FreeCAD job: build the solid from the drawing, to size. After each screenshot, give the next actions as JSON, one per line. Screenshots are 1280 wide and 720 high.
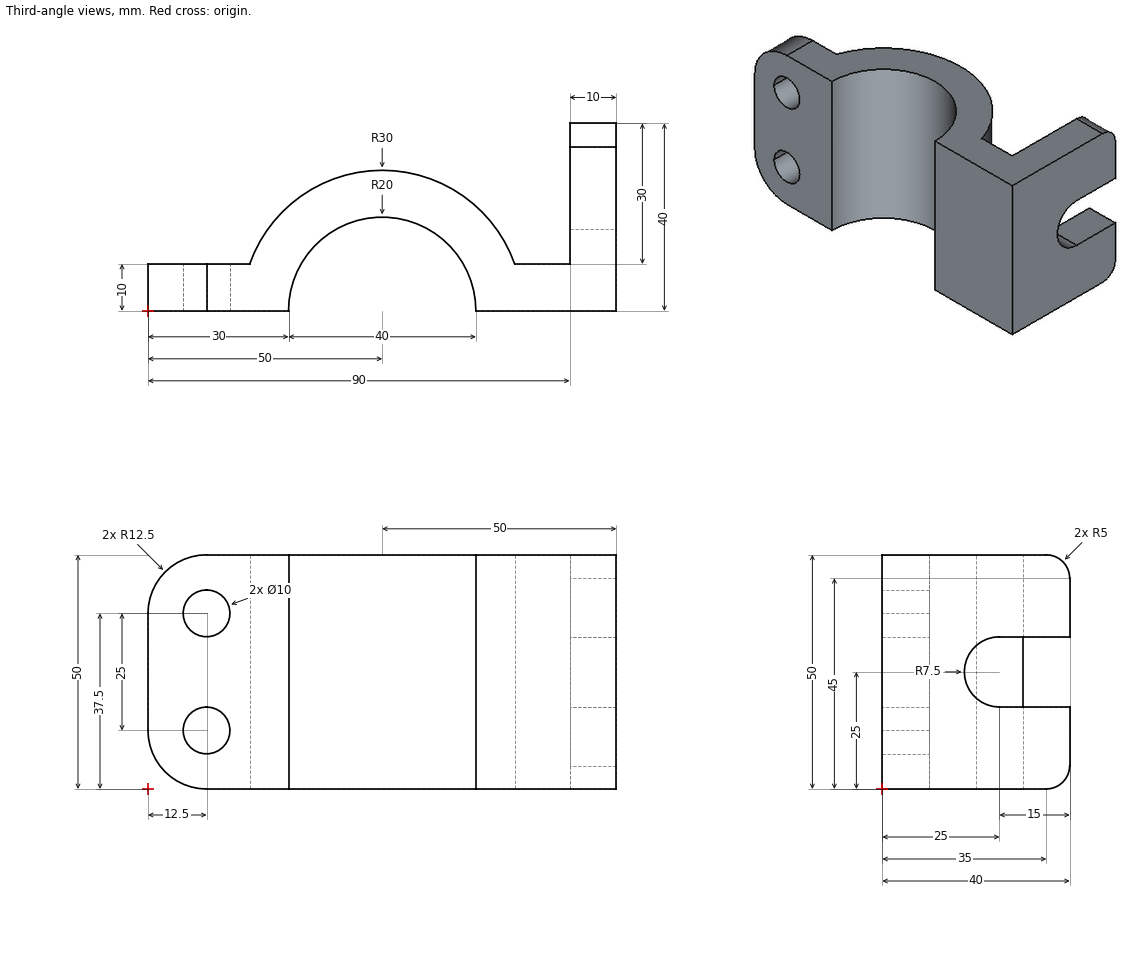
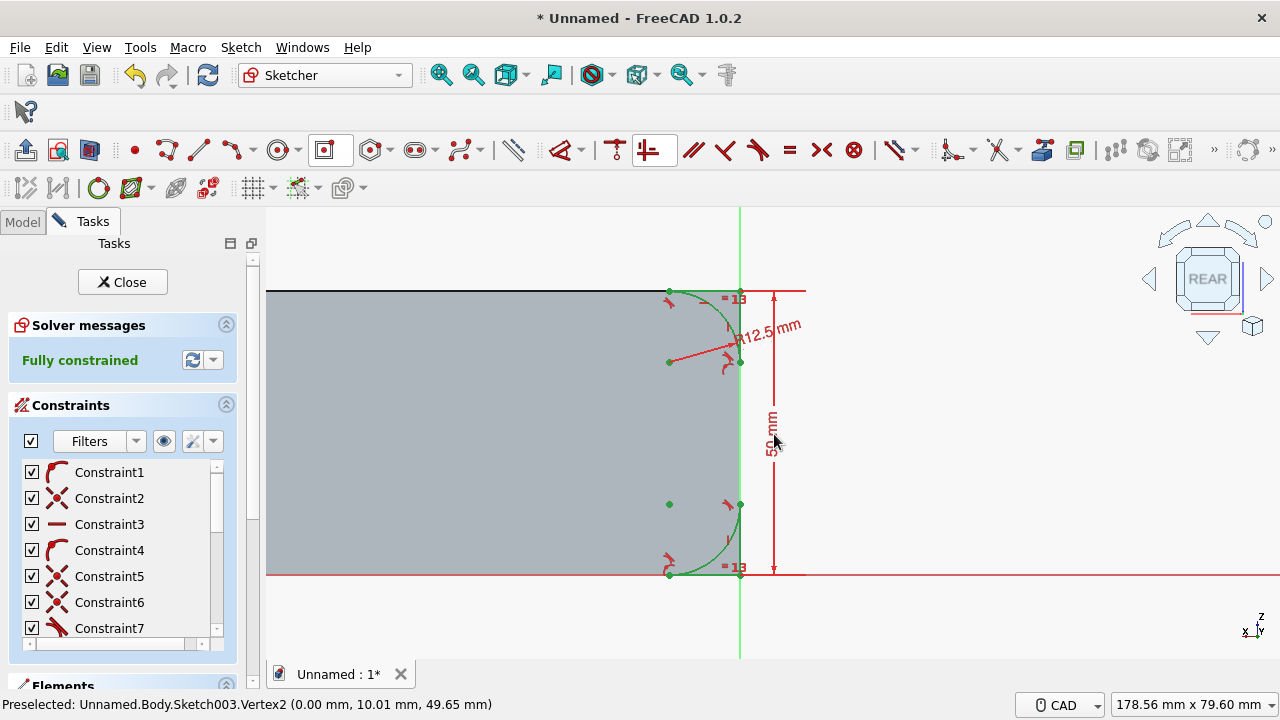
{"action": "left_click", "coordinate": [123, 282]}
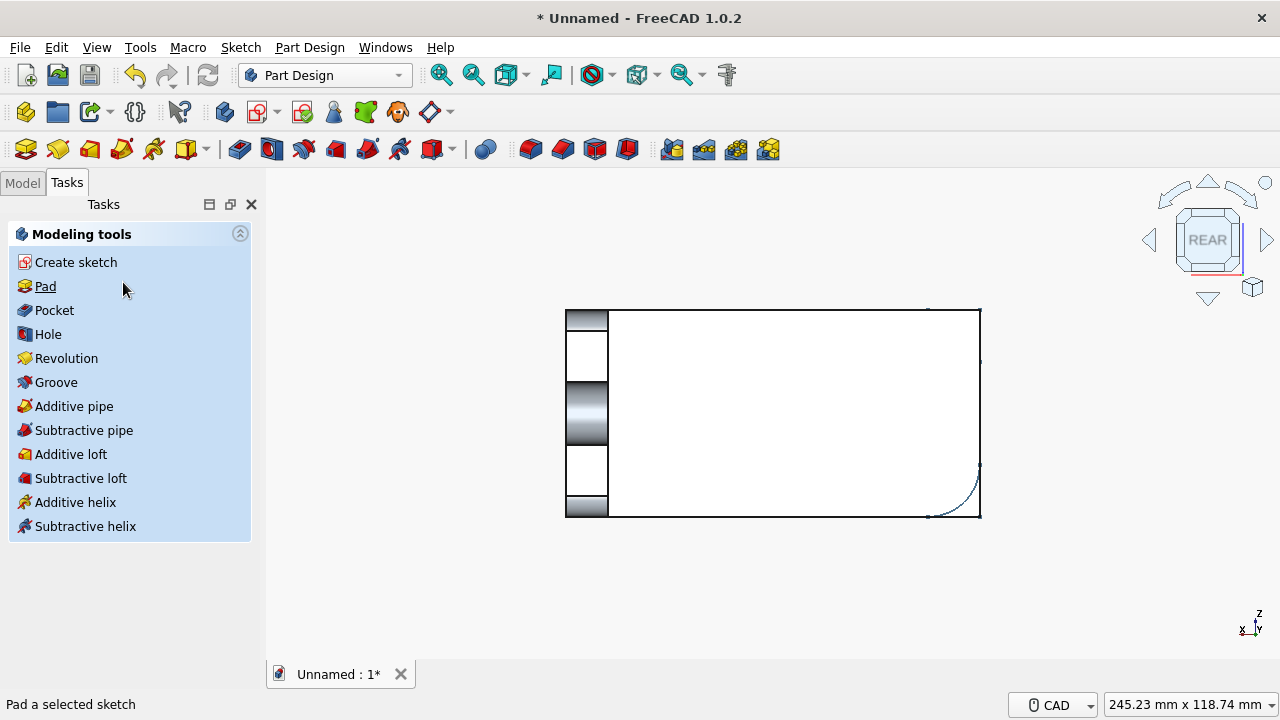
{"action": "left_click", "coordinate": [240, 150]}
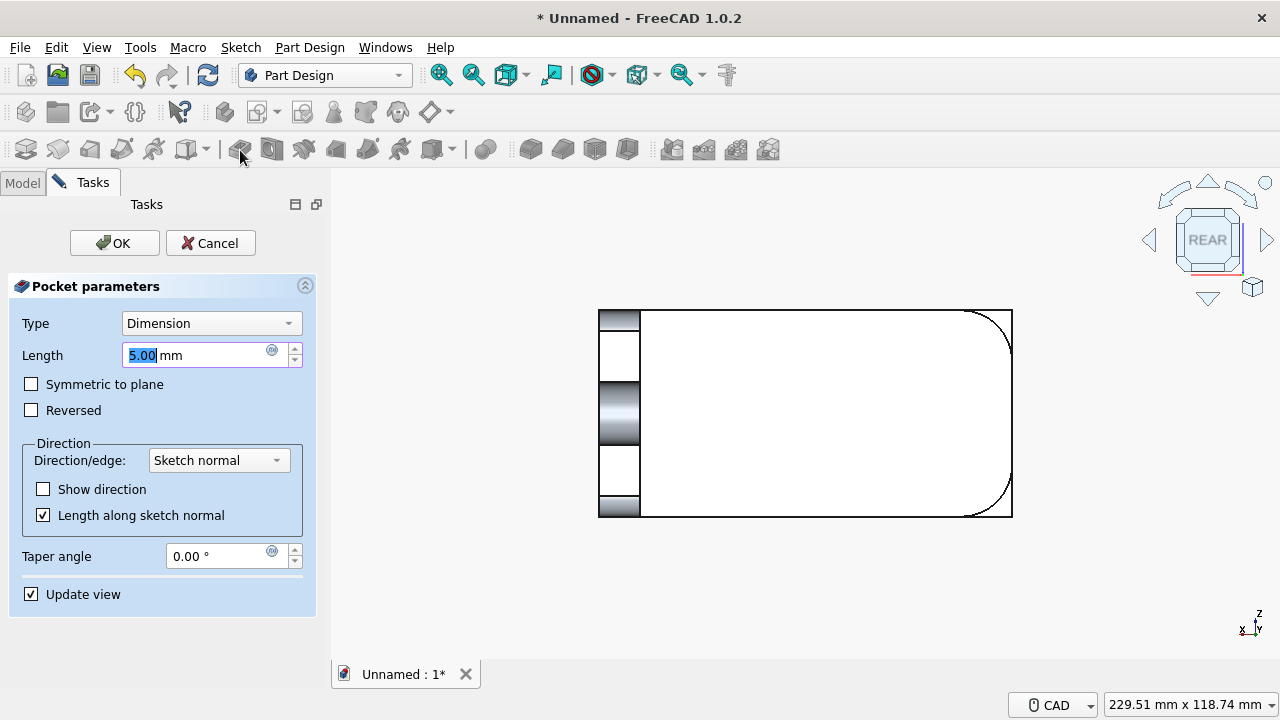
{"action": "type", "text": "50"}
{"action": "key", "text": "Tab"}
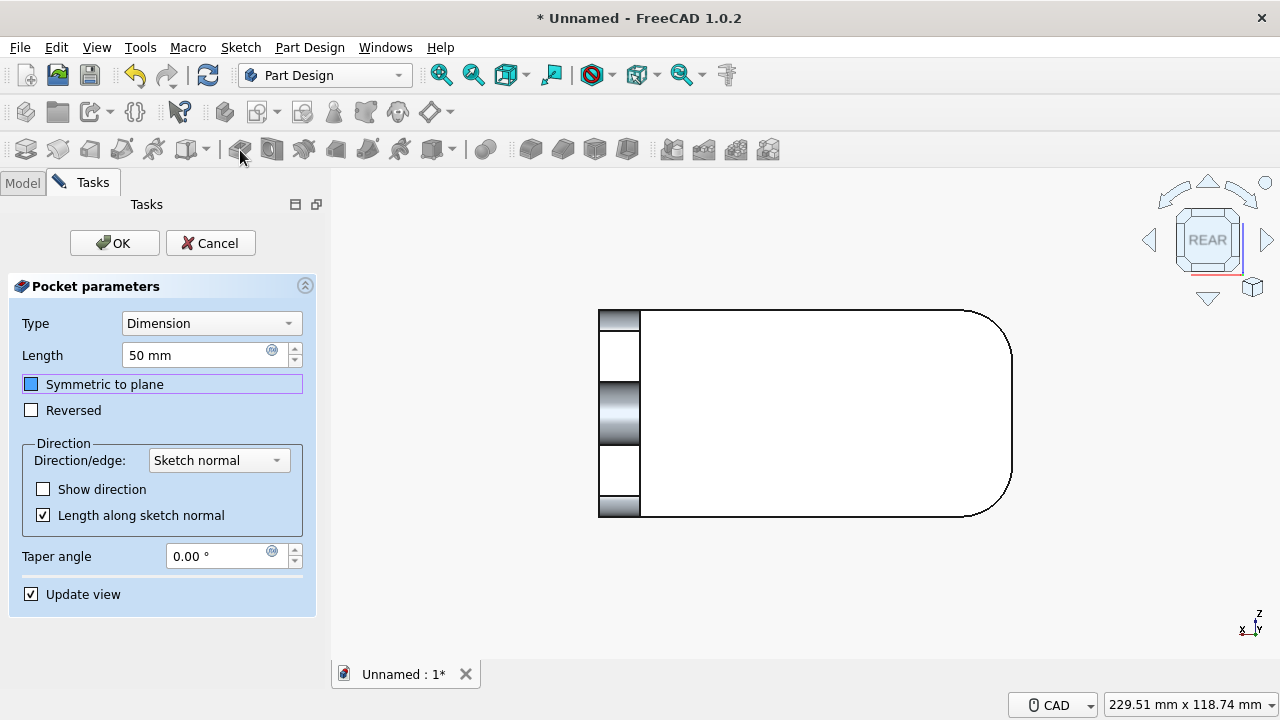
{"action": "left_click", "coordinate": [115, 243]}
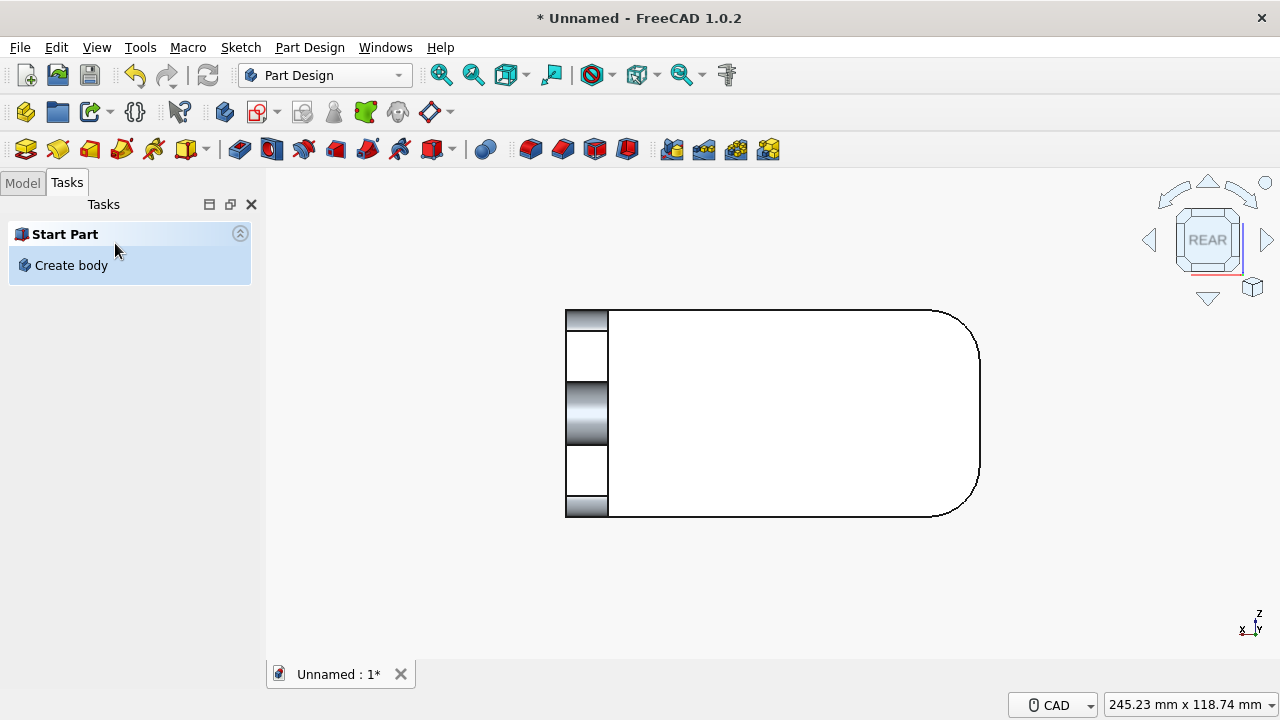
{"action": "left_click", "coordinate": [442, 76]}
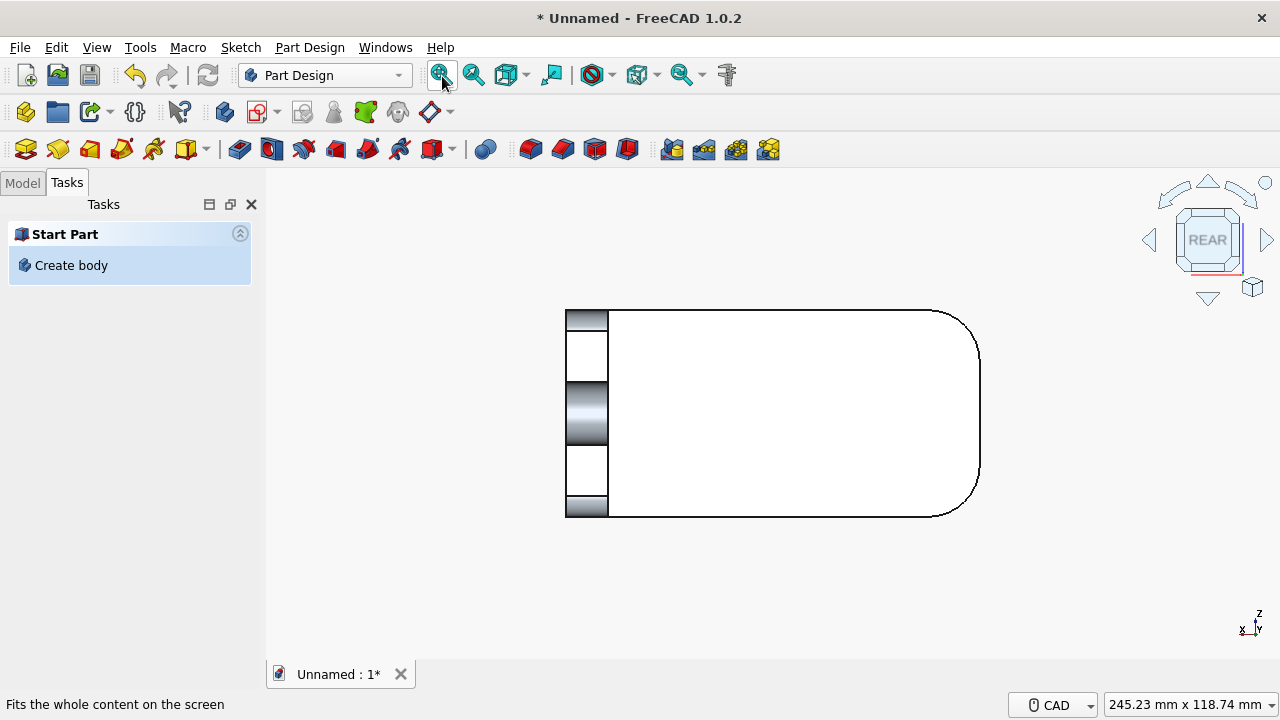
{"action": "key", "text": "0"}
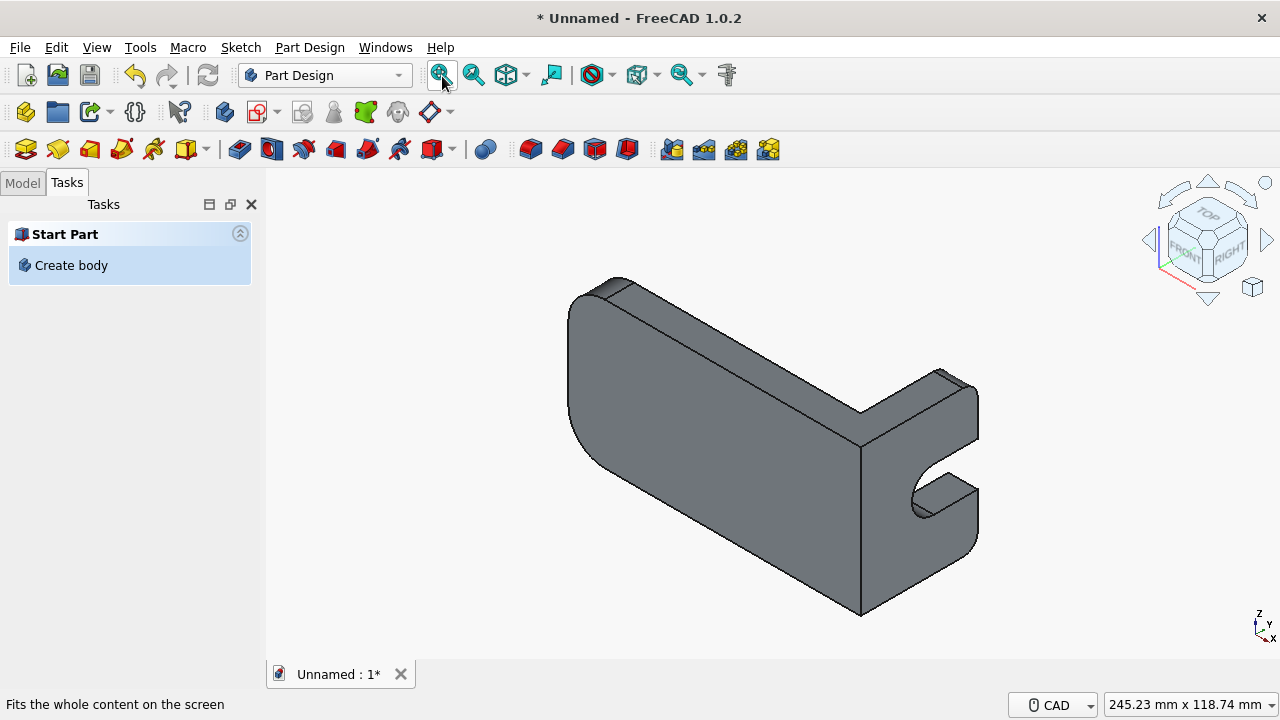
{"action": "left_click", "coordinate": [864, 423]}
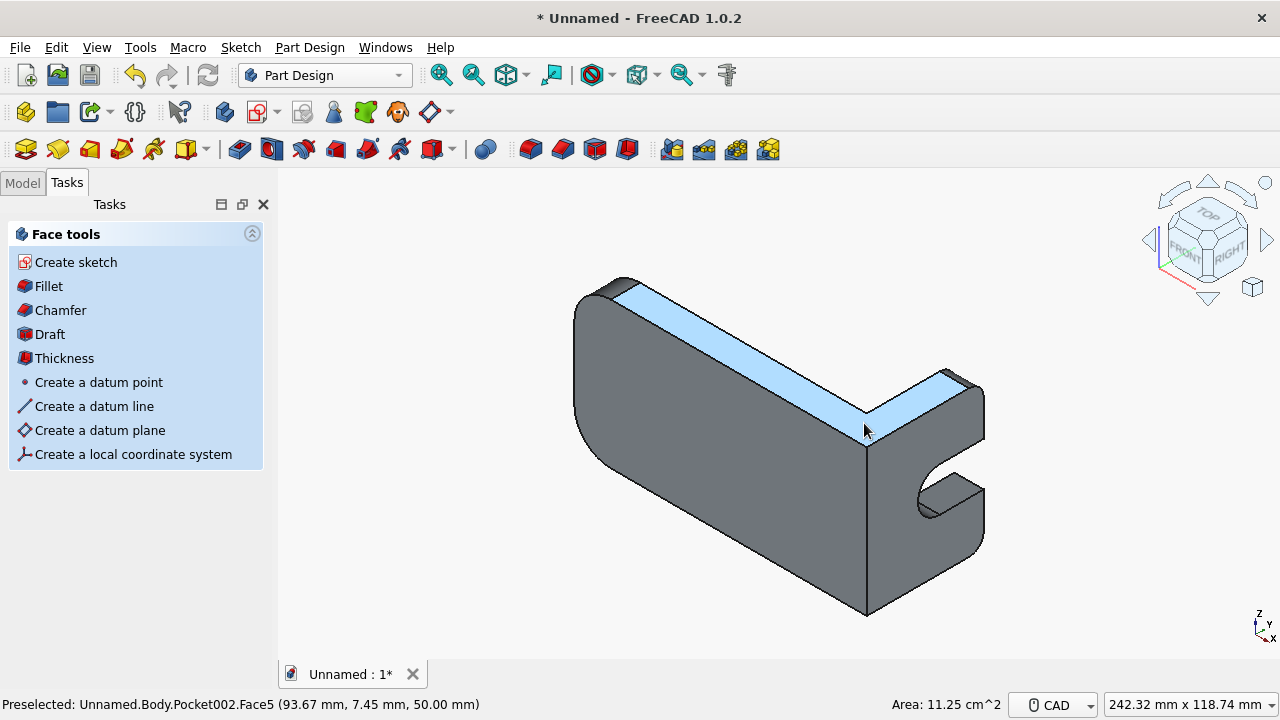
{"action": "left_click", "coordinate": [258, 112]}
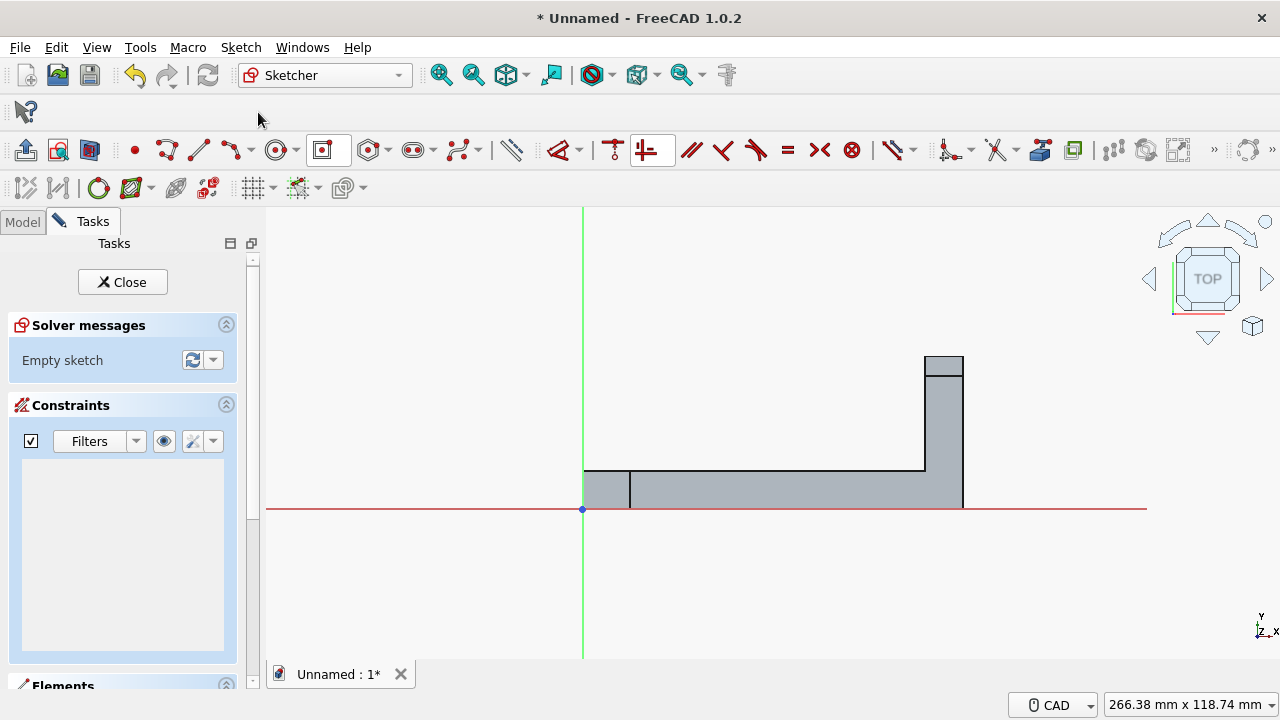
{"action": "scroll", "coordinate": [765, 475], "scroll_direction": "up", "scroll_amount": 3}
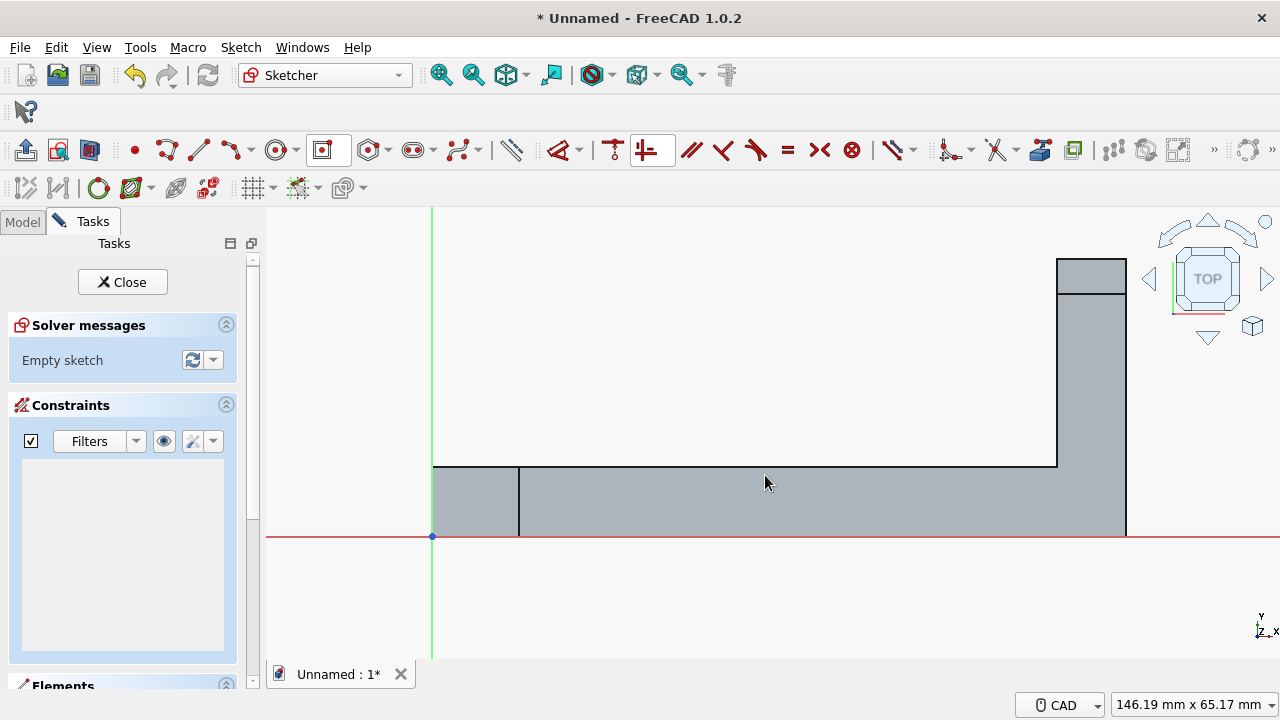
{"action": "left_click", "coordinate": [200, 150]}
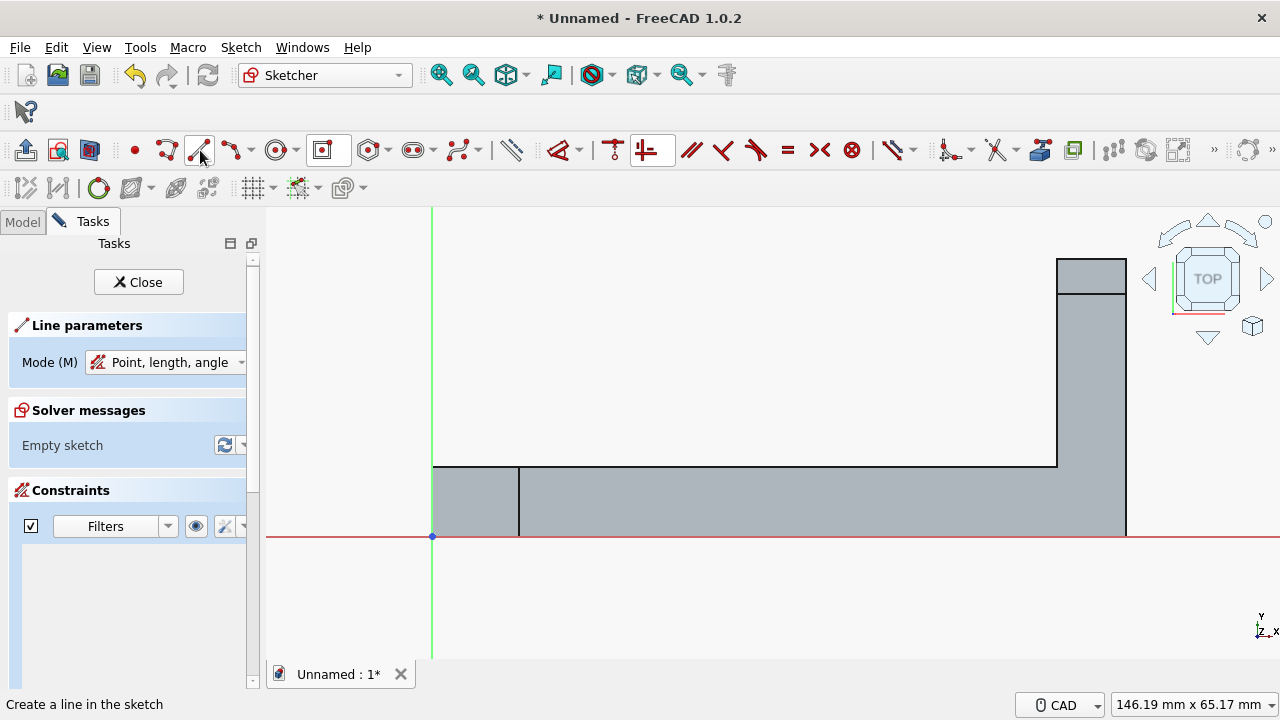
{"action": "left_click", "coordinate": [583, 467]}
{"action": "left_click", "coordinate": [975, 467]}